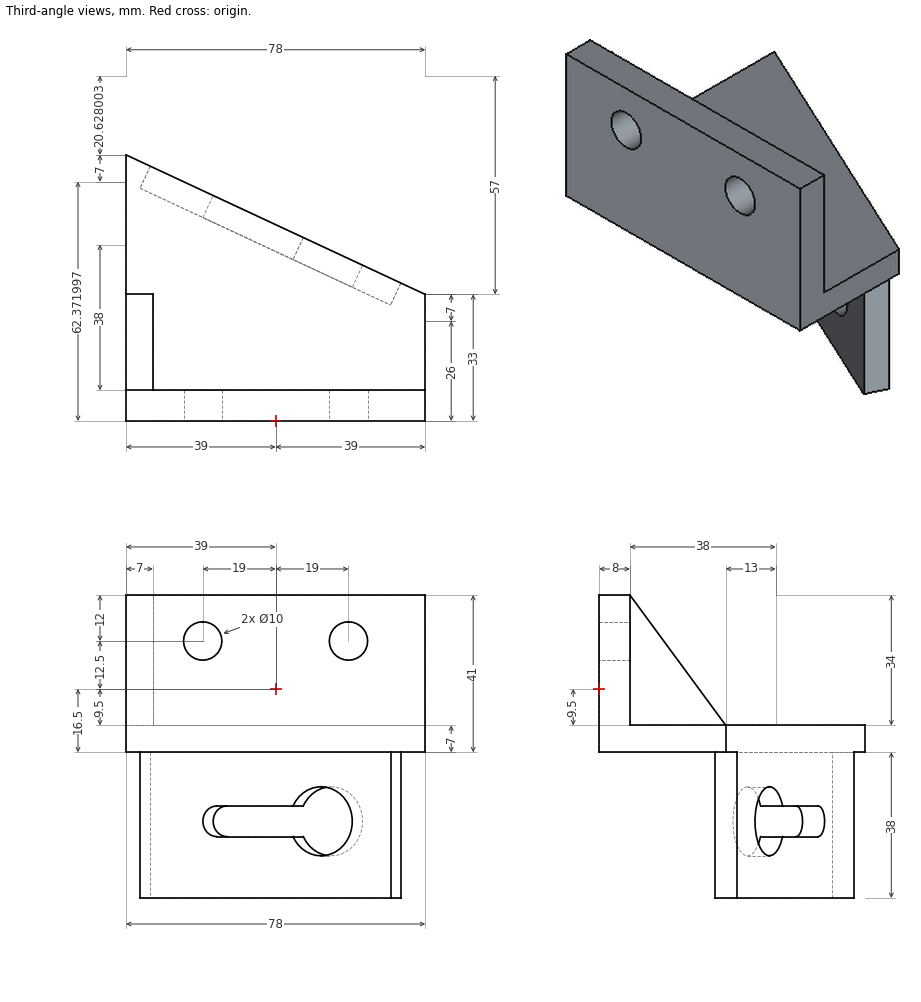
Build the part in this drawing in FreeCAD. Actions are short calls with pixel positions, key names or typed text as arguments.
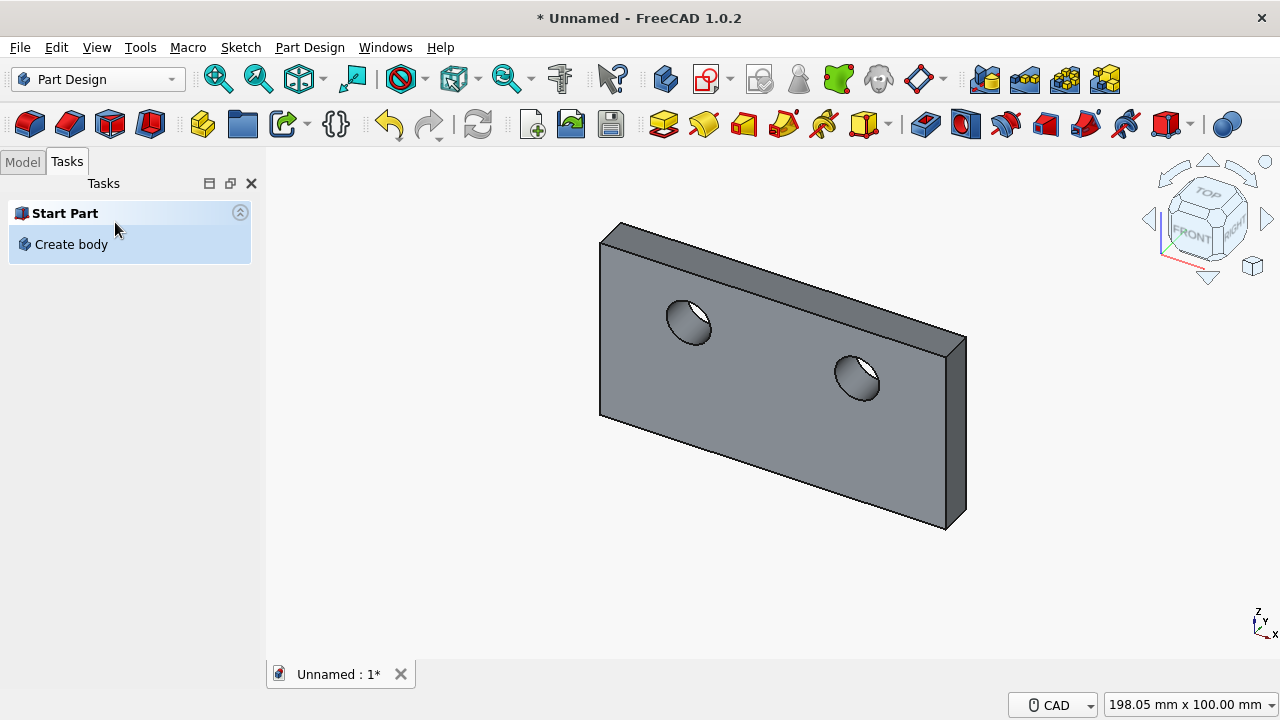
key(4)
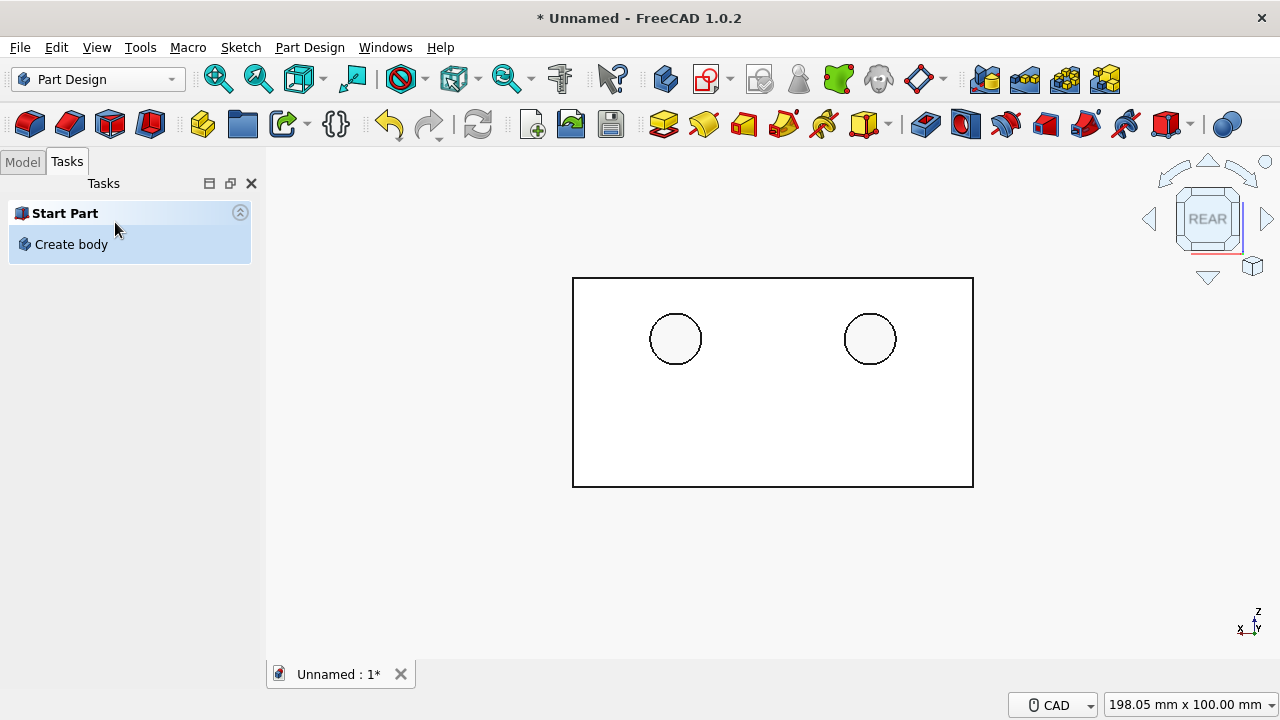
click(220, 80)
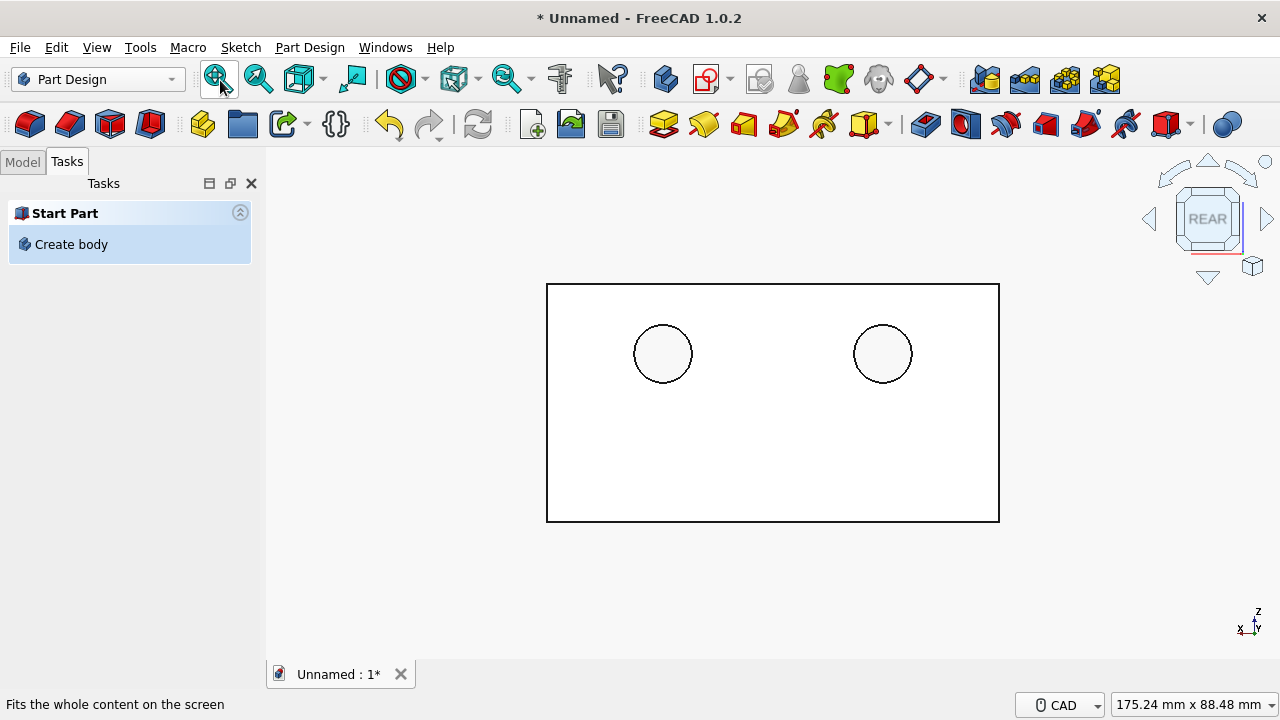
click(773, 402)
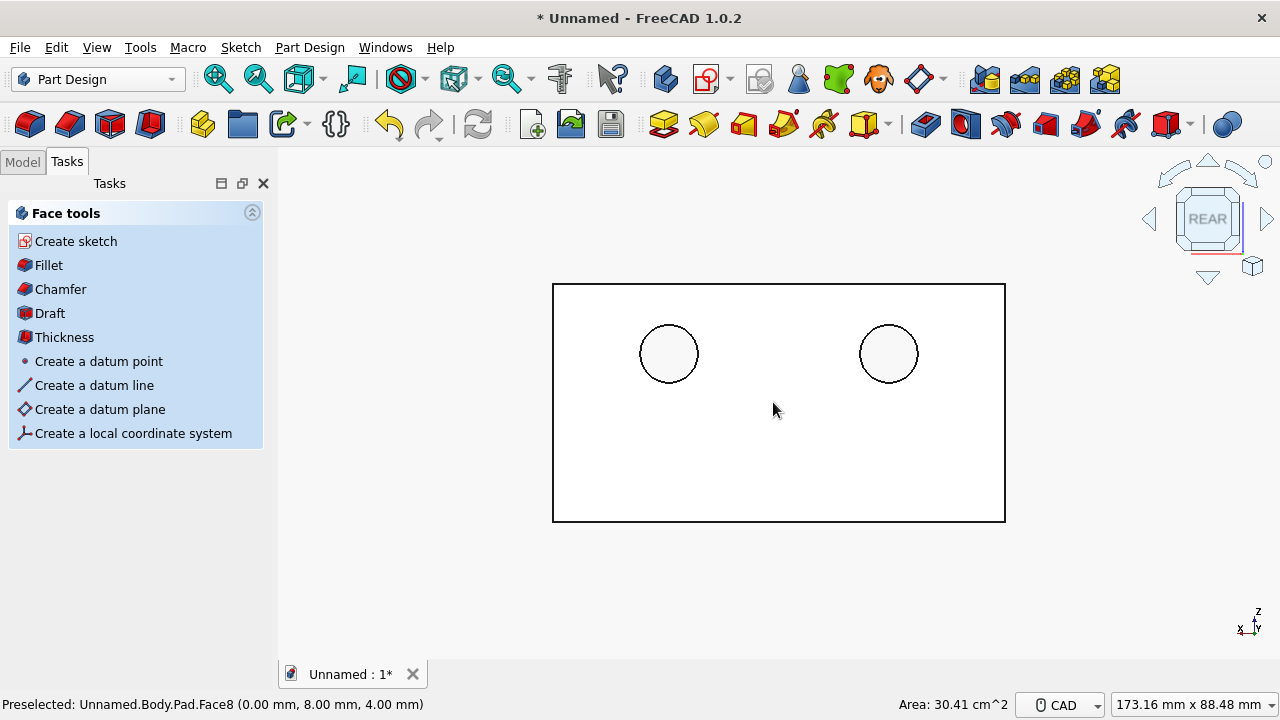
click(706, 80)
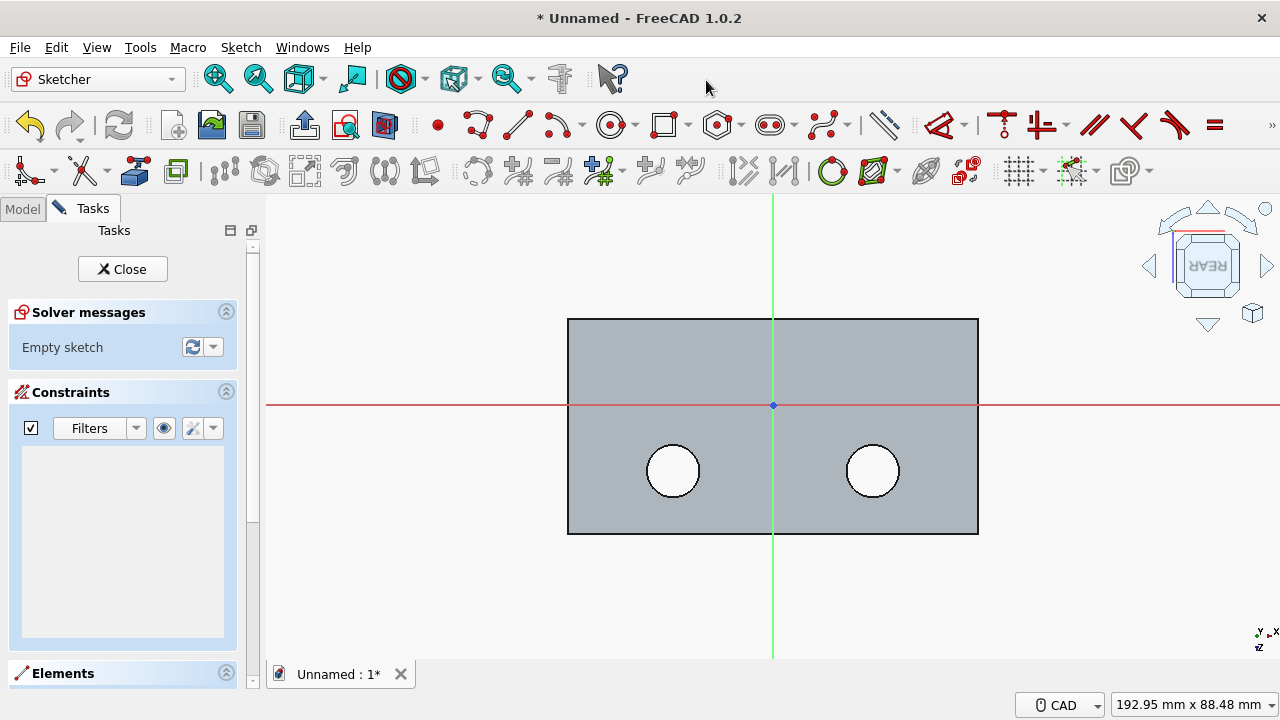
click(664, 126)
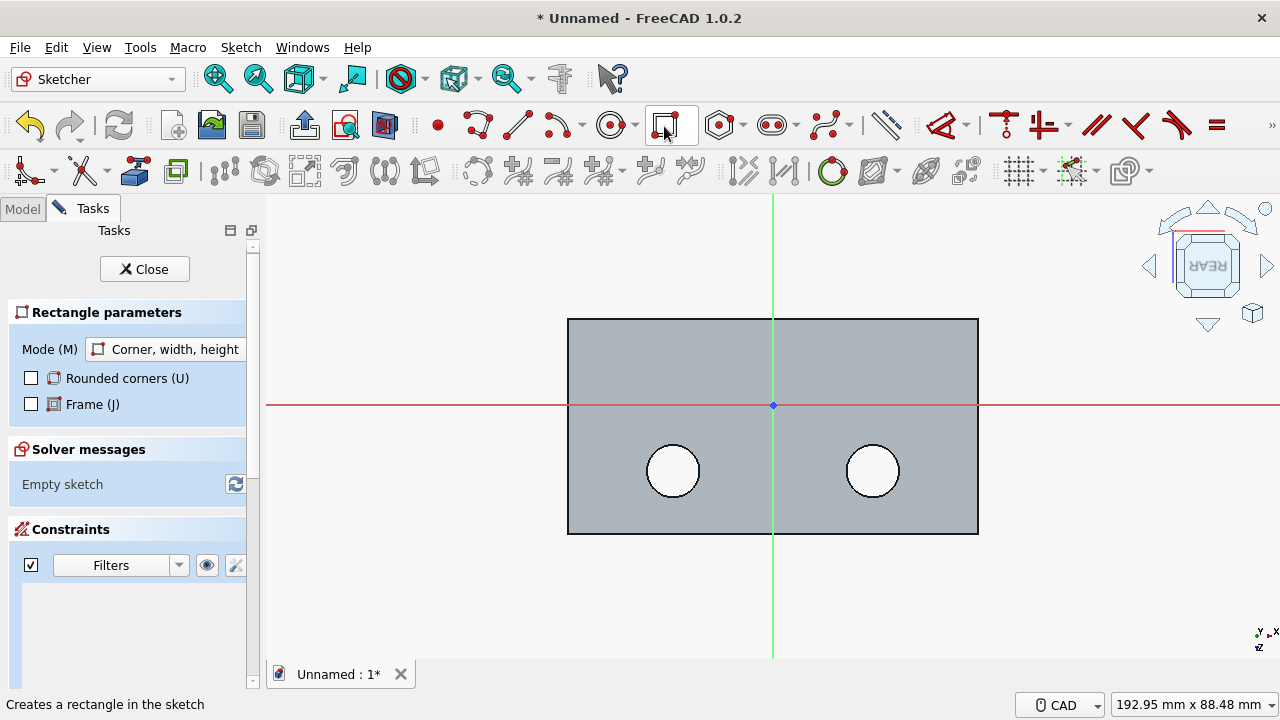
click(568, 319)
move(605, 534)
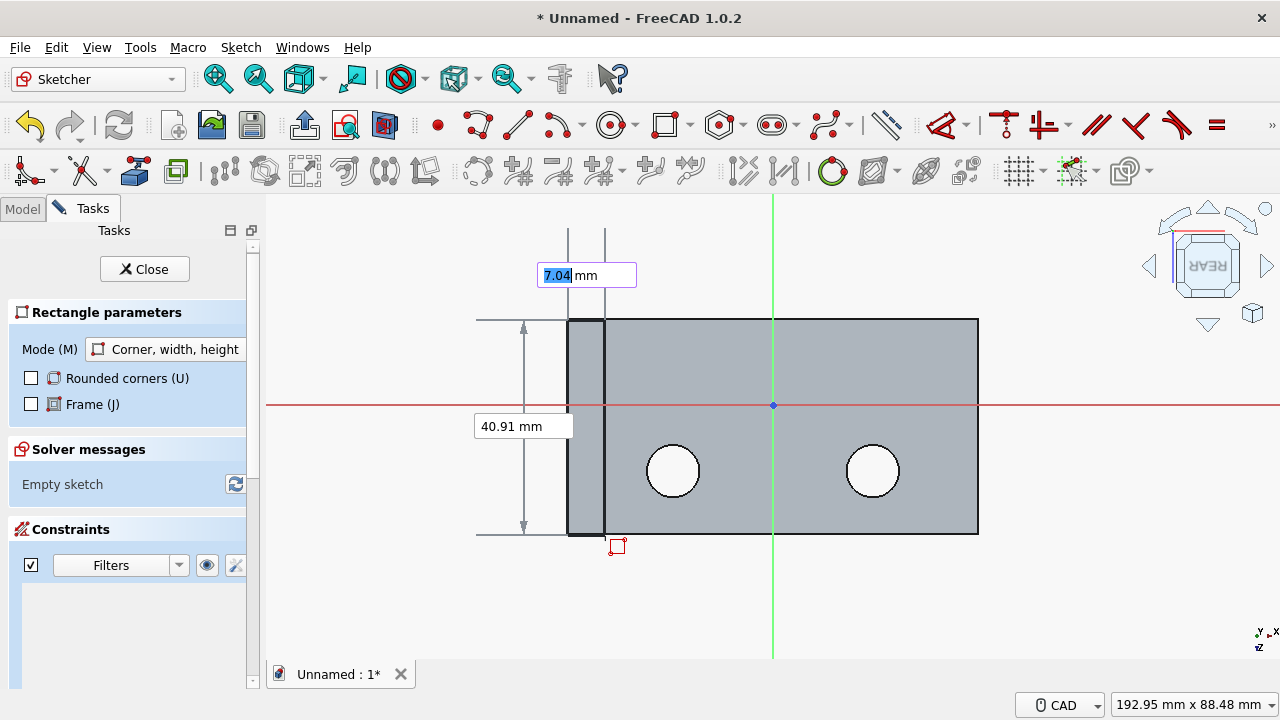
text(7)
key(Tab)
text(41)
key(Return)
key(Escape)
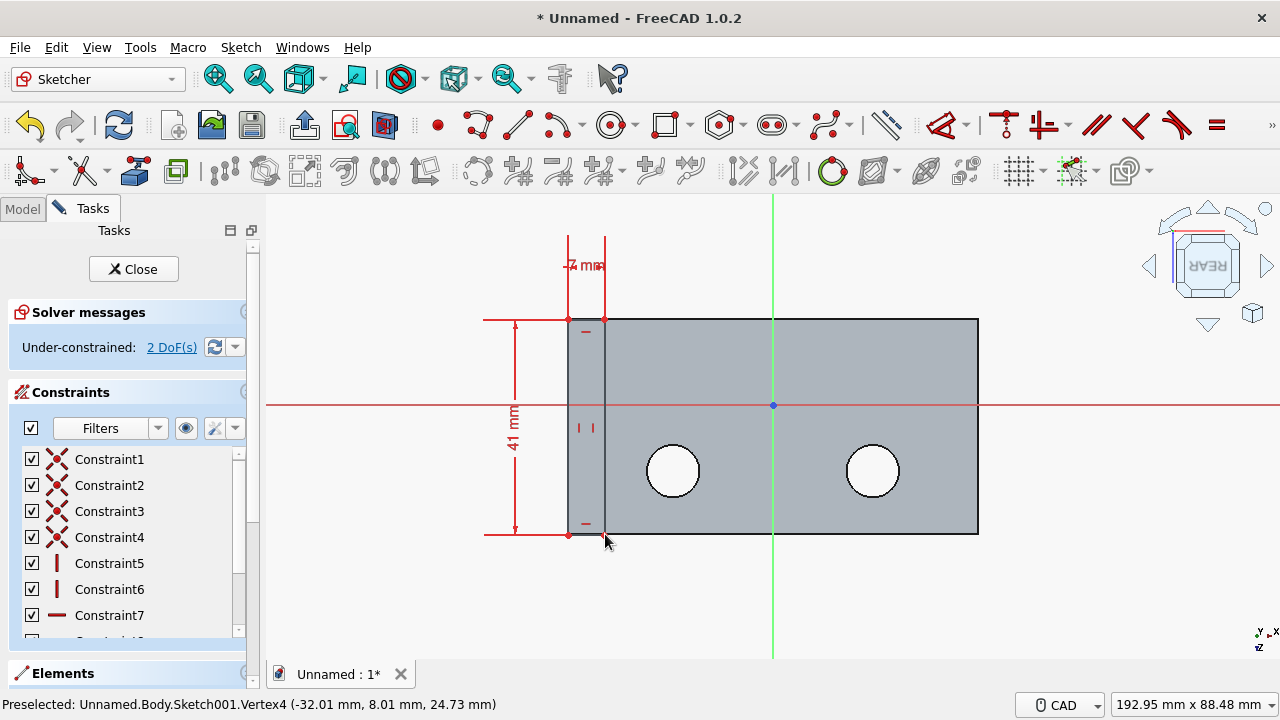
click(942, 126)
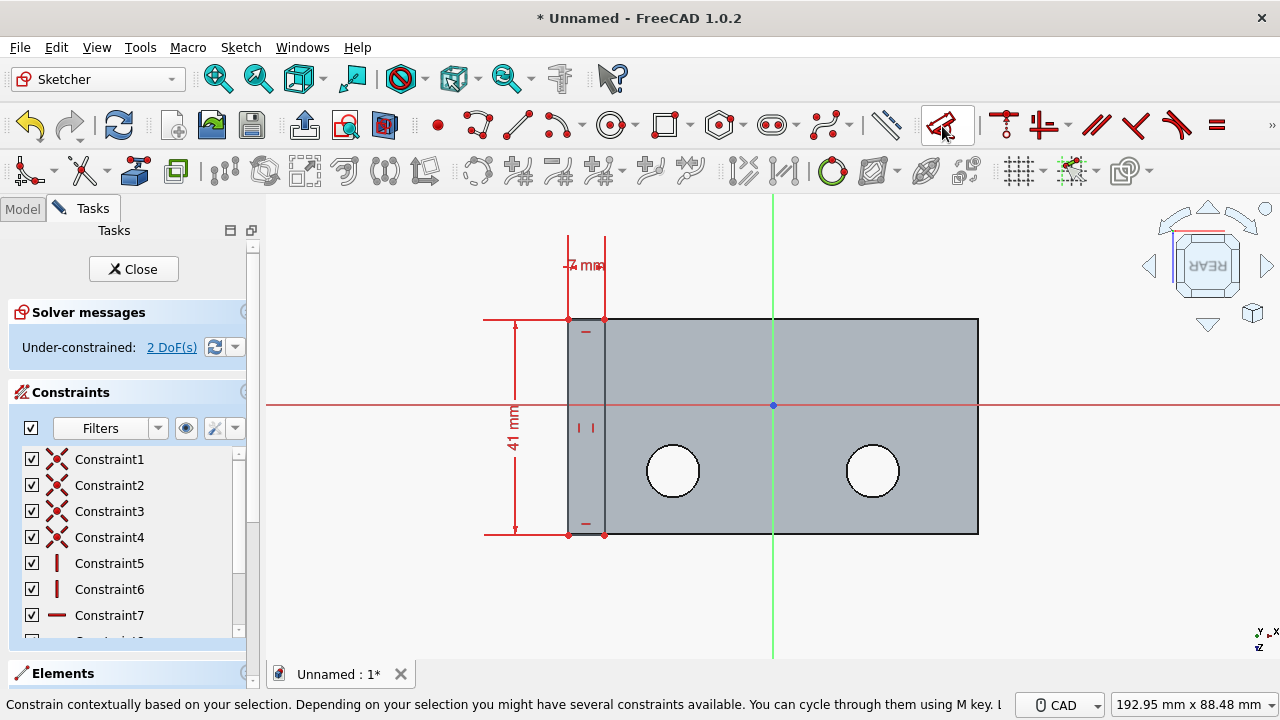
click(568, 320)
click(670, 286)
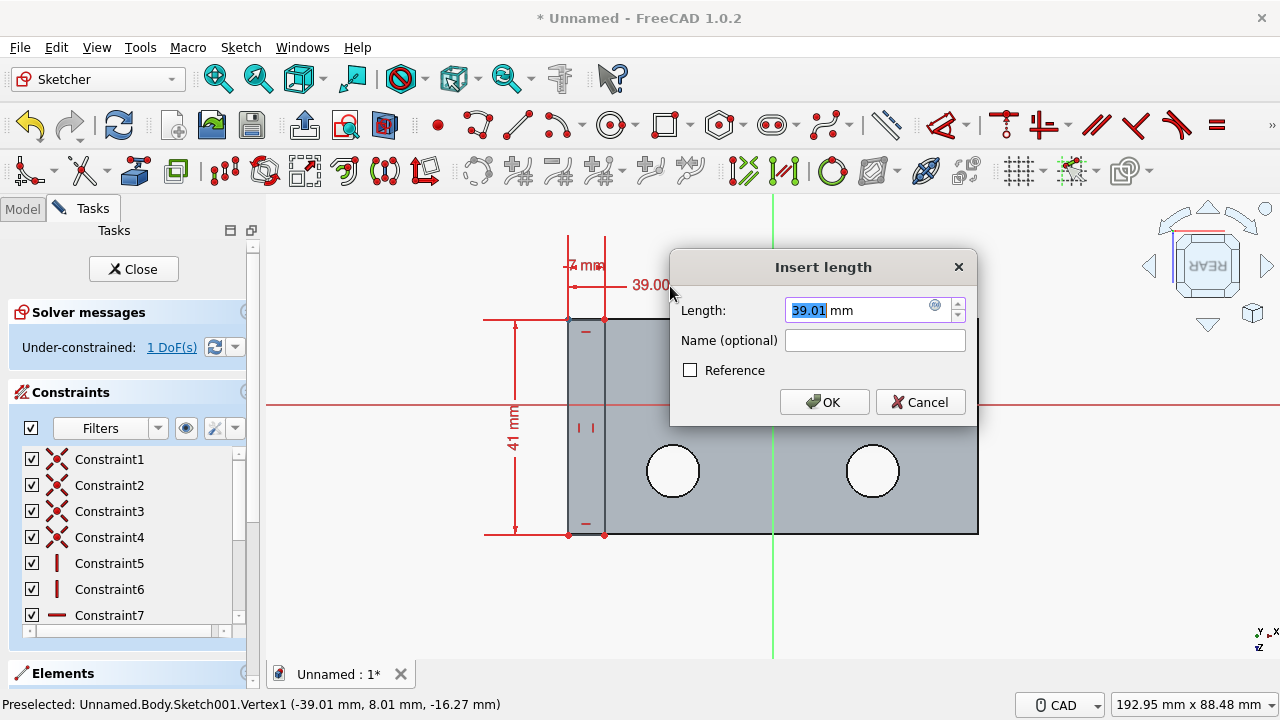
text(39)
key(Return)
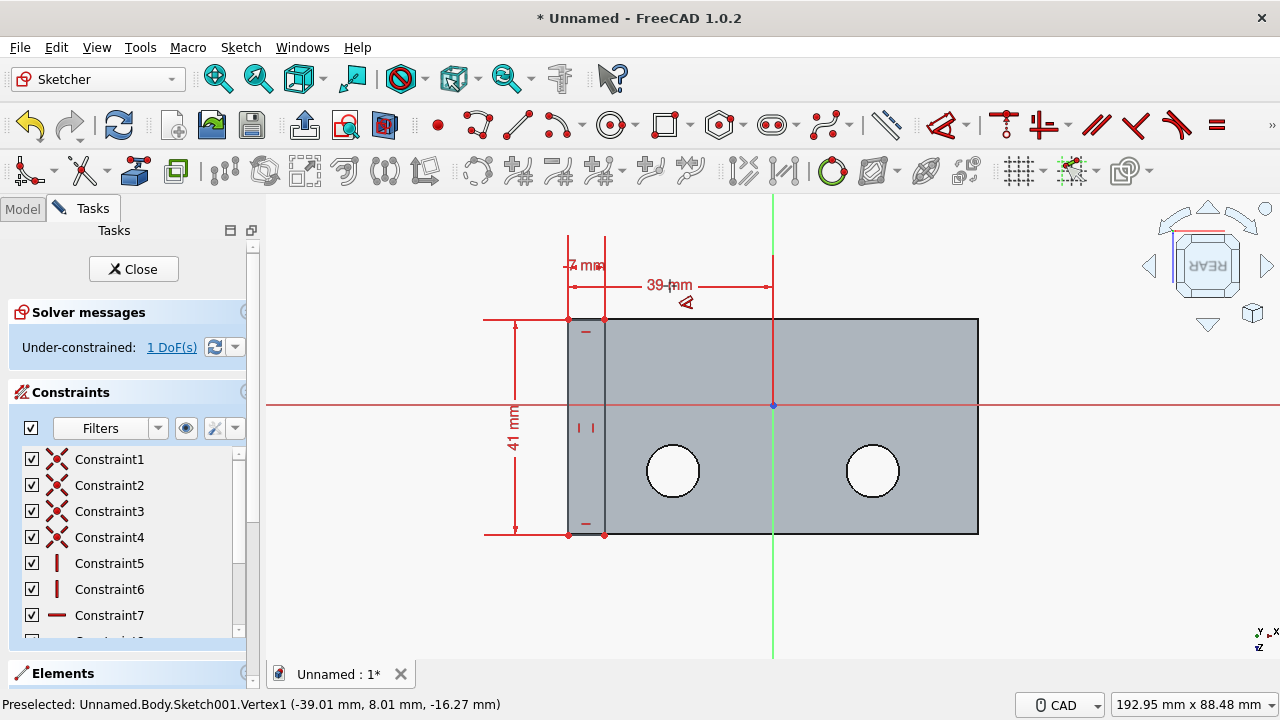
click(568, 320)
click(807, 363)